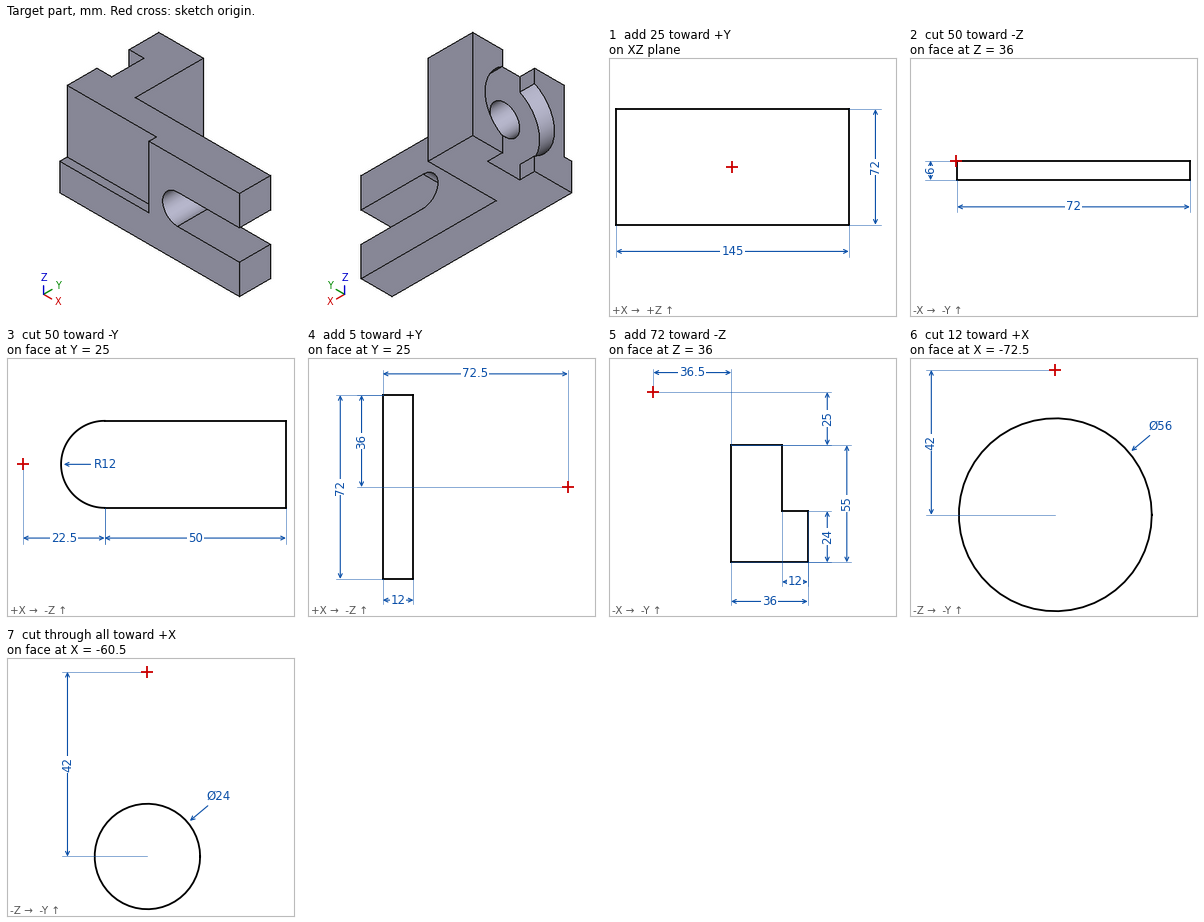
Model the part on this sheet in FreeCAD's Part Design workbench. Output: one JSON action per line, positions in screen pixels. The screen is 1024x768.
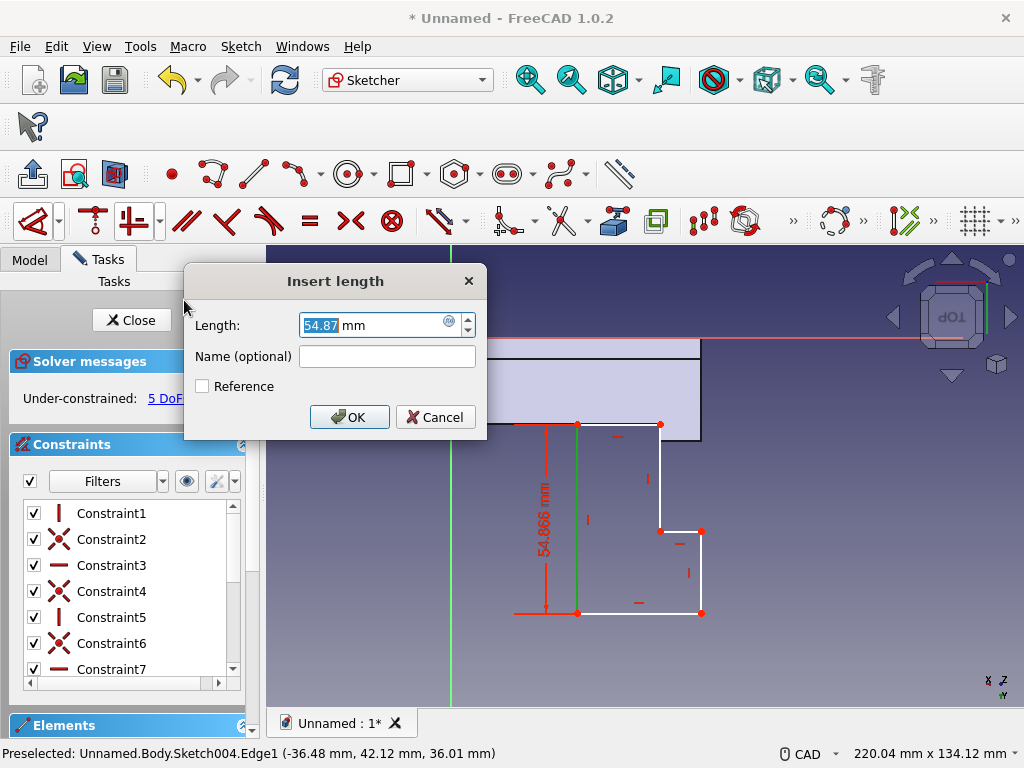
{"action": "type", "text": "55"}
{"action": "key", "text": "Return"}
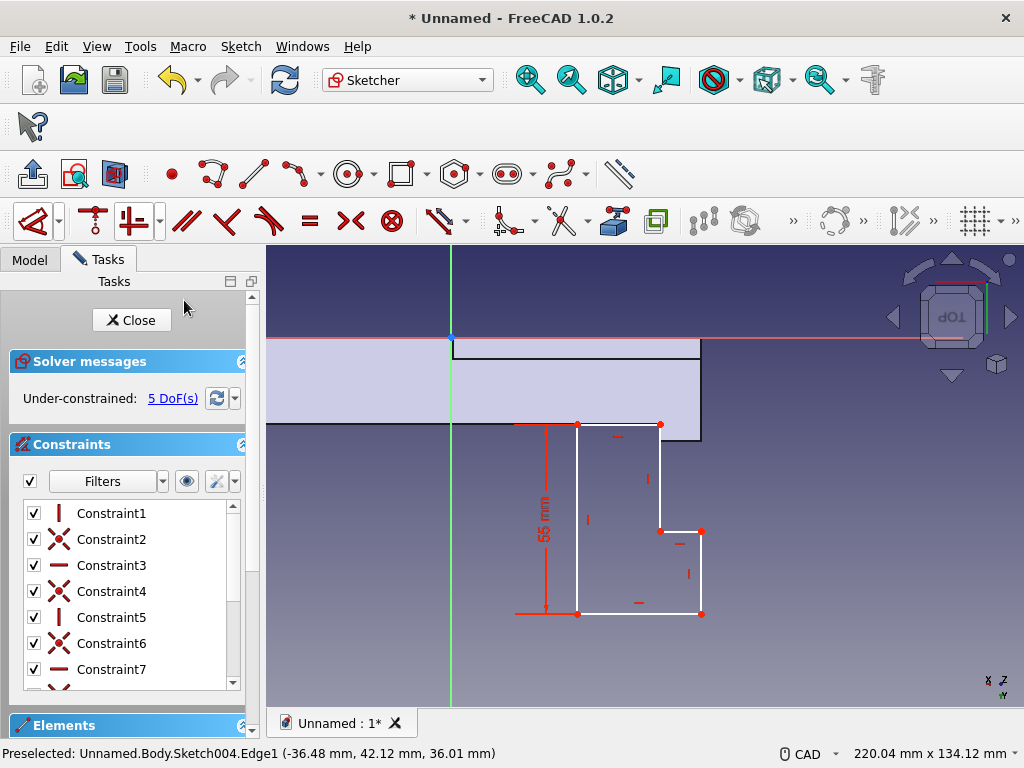
{"action": "left_click", "coordinate": [614, 614]}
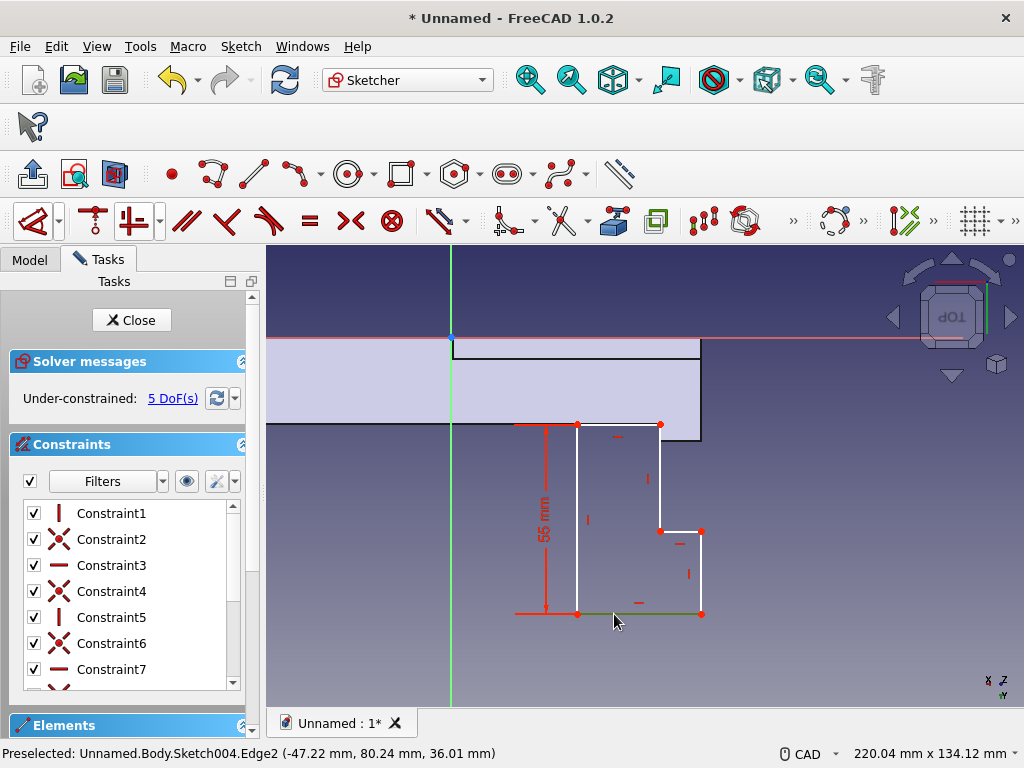
{"action": "key", "text": "l"}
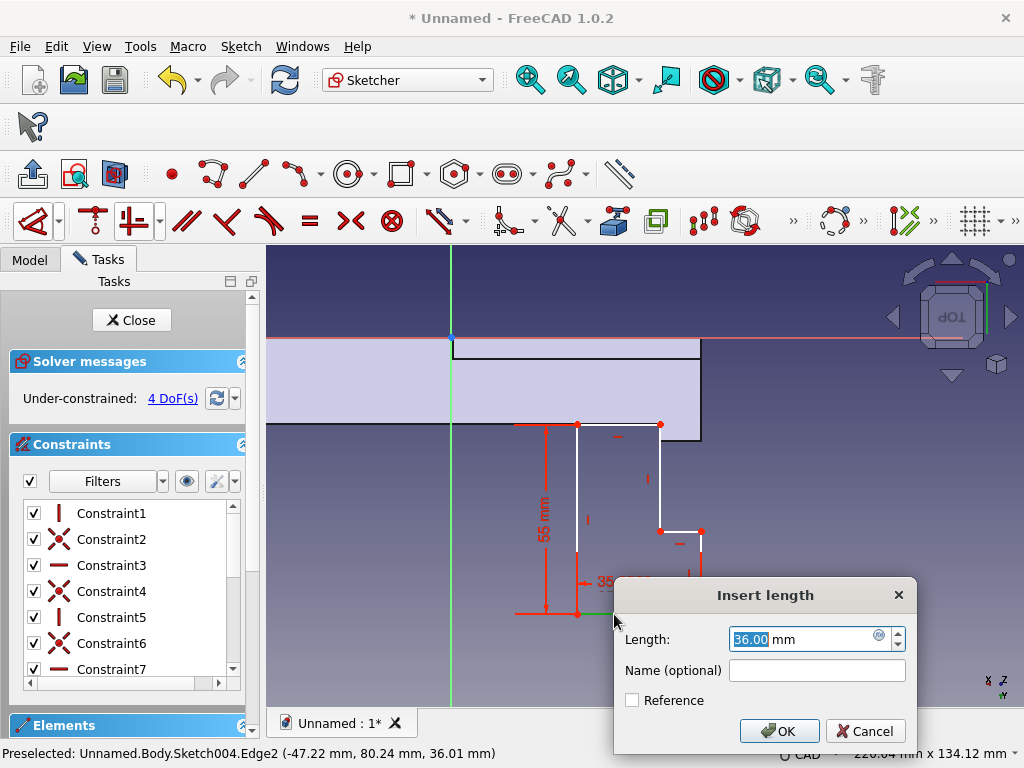
{"action": "type", "text": "36"}
{"action": "key", "text": "Return"}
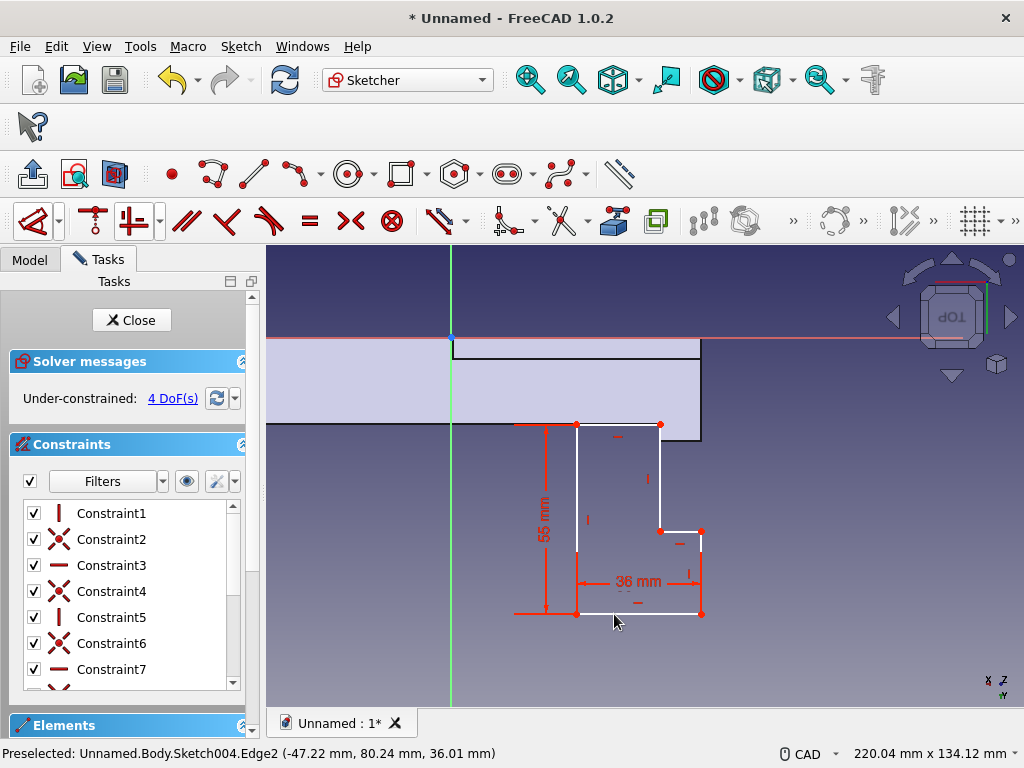
{"action": "left_click", "coordinate": [701, 590]}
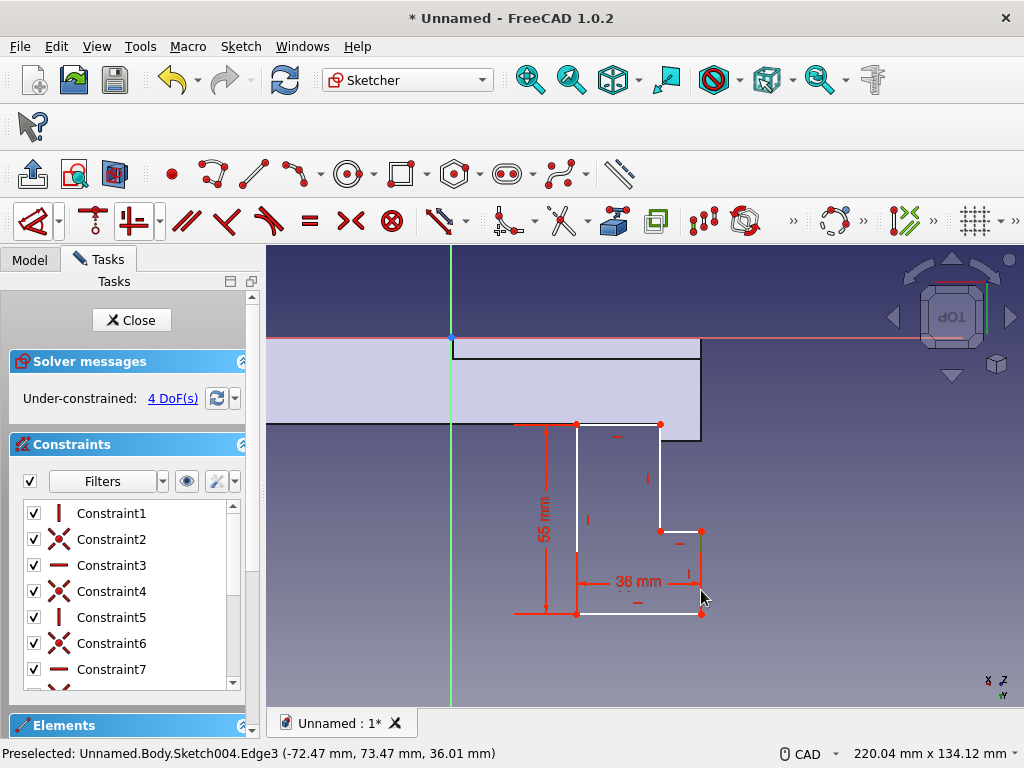
{"action": "key", "text": "i"}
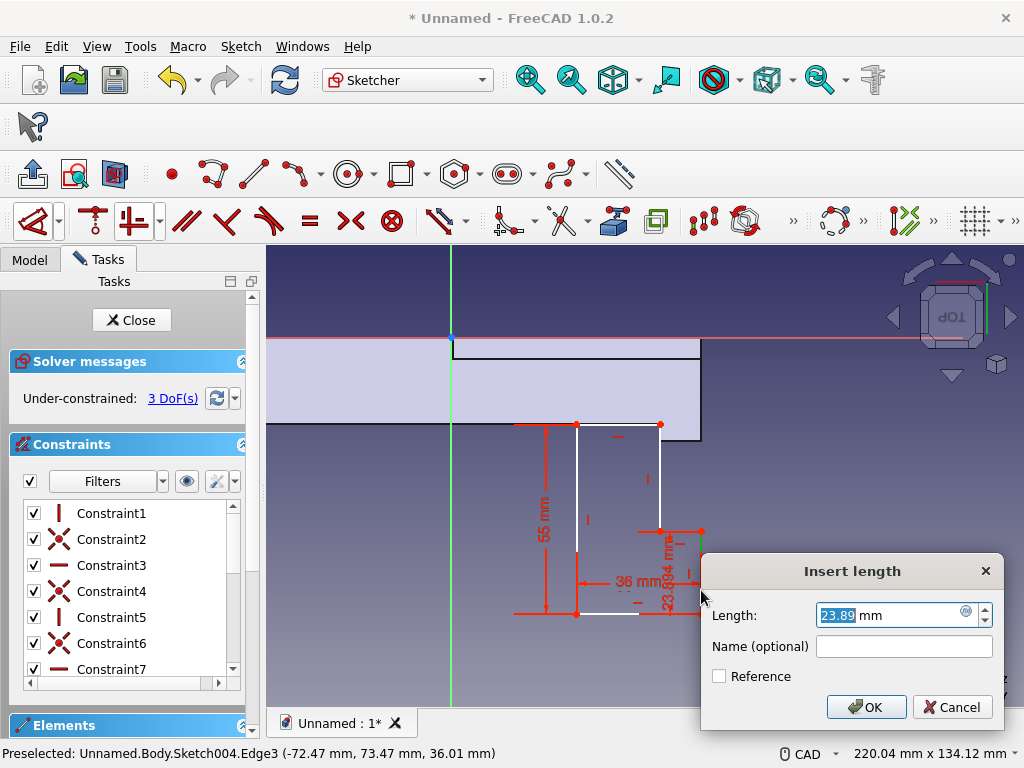
{"action": "type", "text": "24"}
{"action": "key", "text": "Return"}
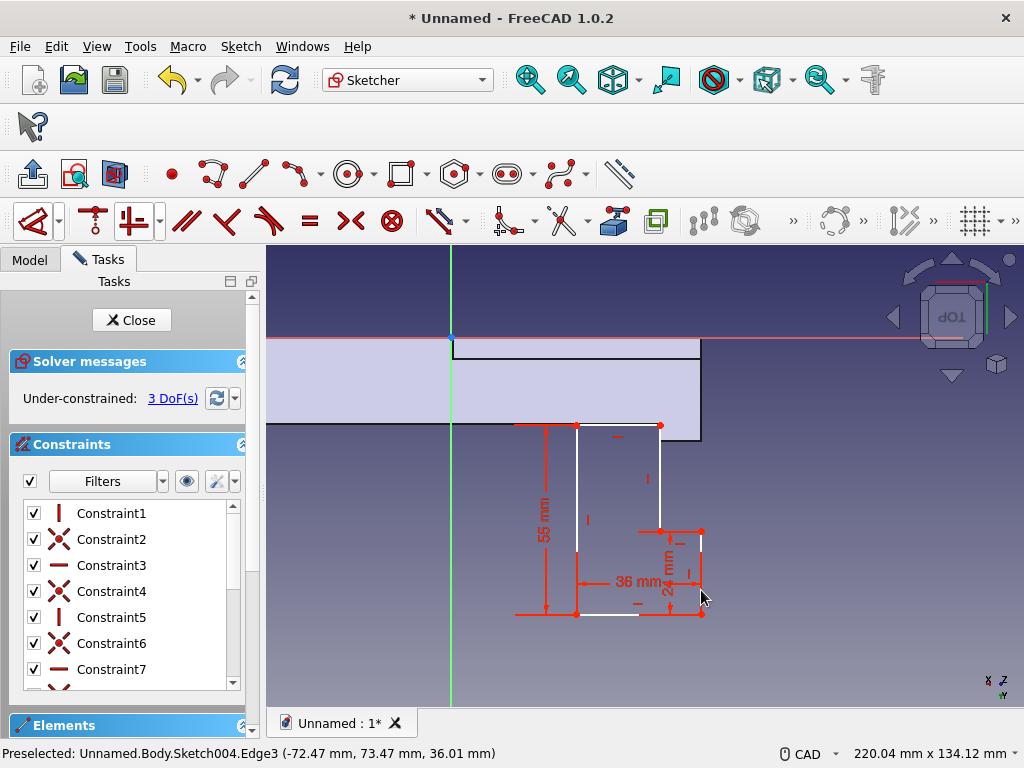
{"action": "left_click", "coordinate": [689, 532]}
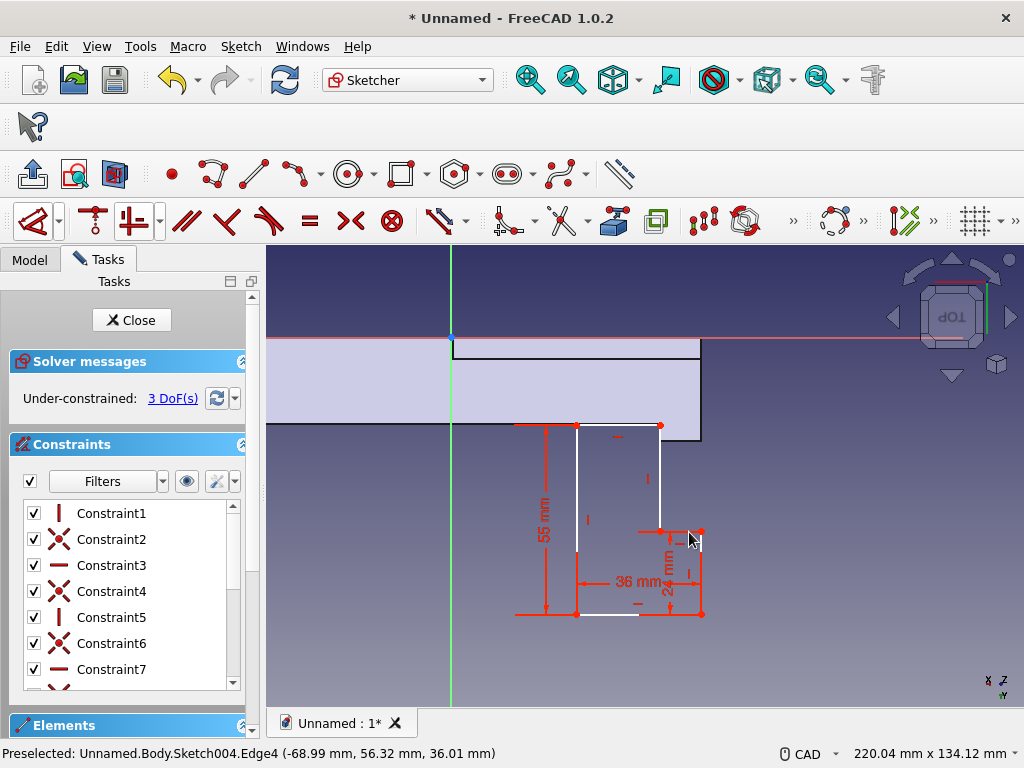
{"action": "left_click", "coordinate": [58, 222]}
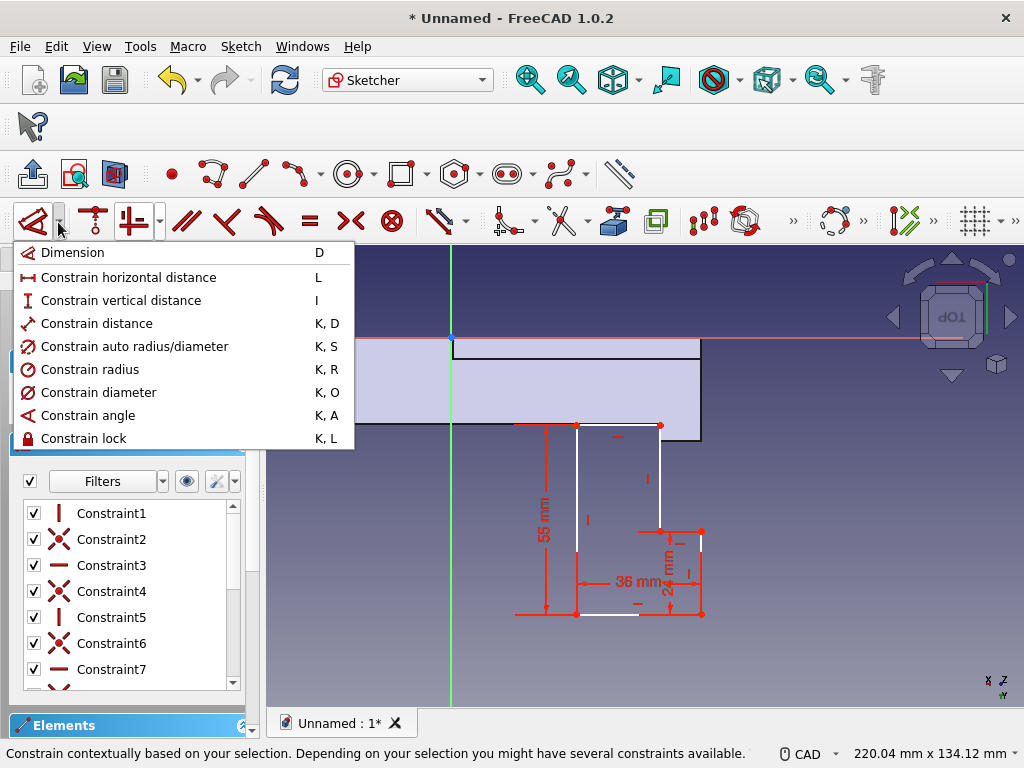
{"action": "left_click", "coordinate": [184, 278]}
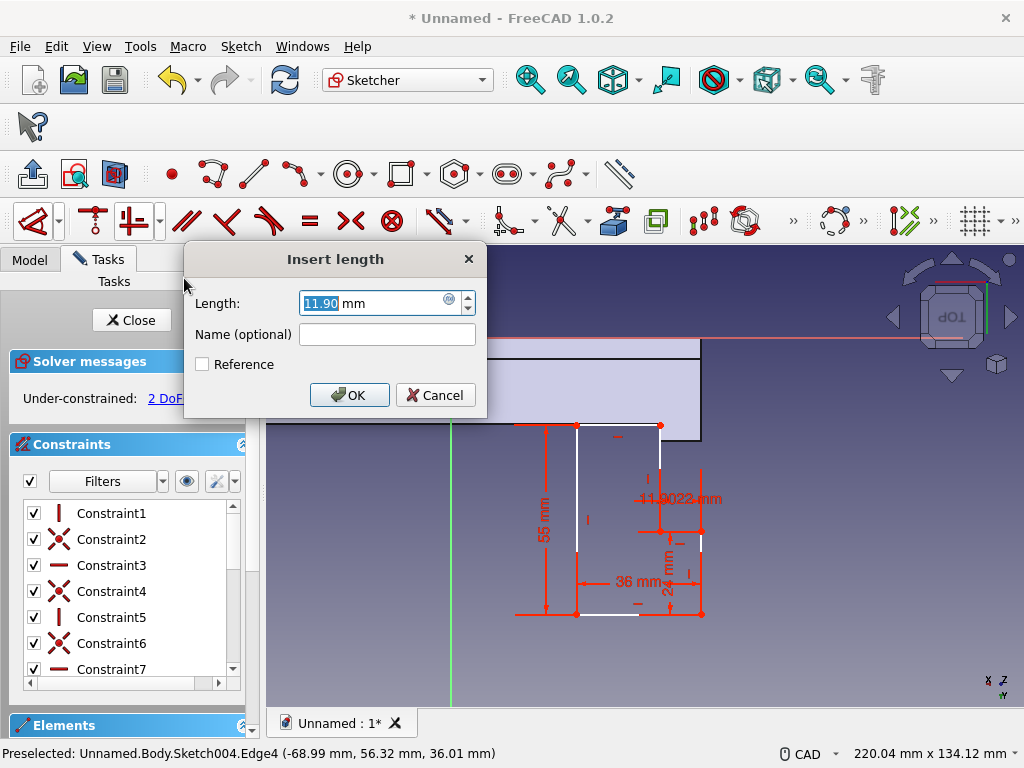
{"action": "type", "text": "12"}
{"action": "key", "text": "Return"}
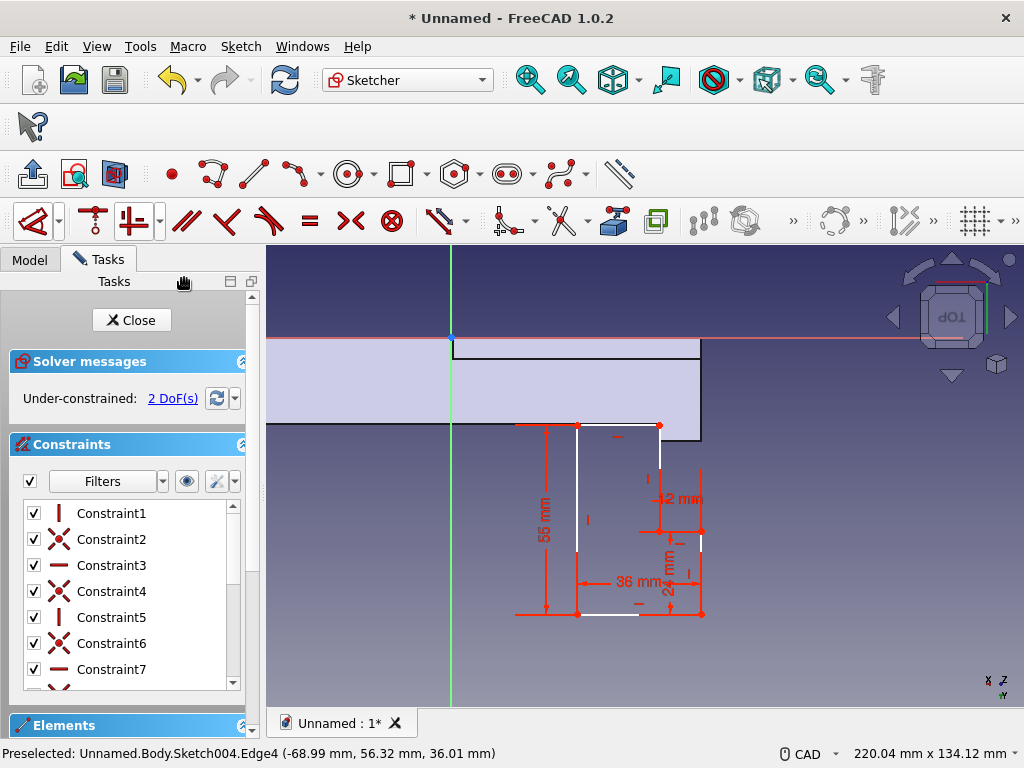
{"action": "left_click", "coordinate": [577, 425]}